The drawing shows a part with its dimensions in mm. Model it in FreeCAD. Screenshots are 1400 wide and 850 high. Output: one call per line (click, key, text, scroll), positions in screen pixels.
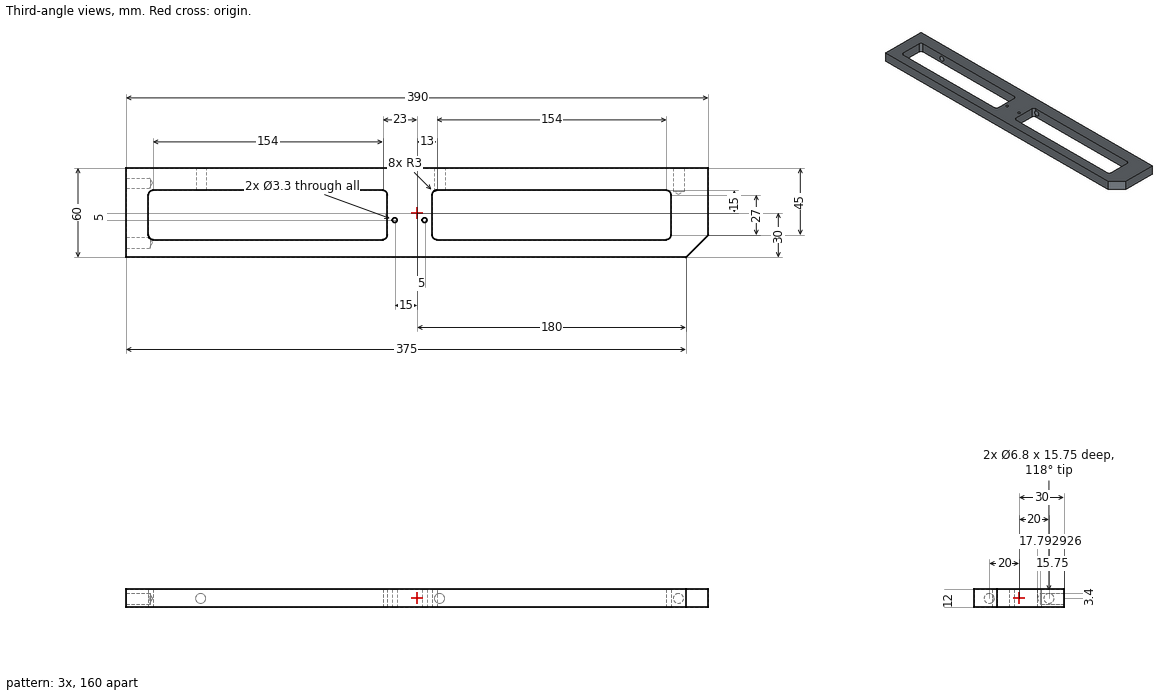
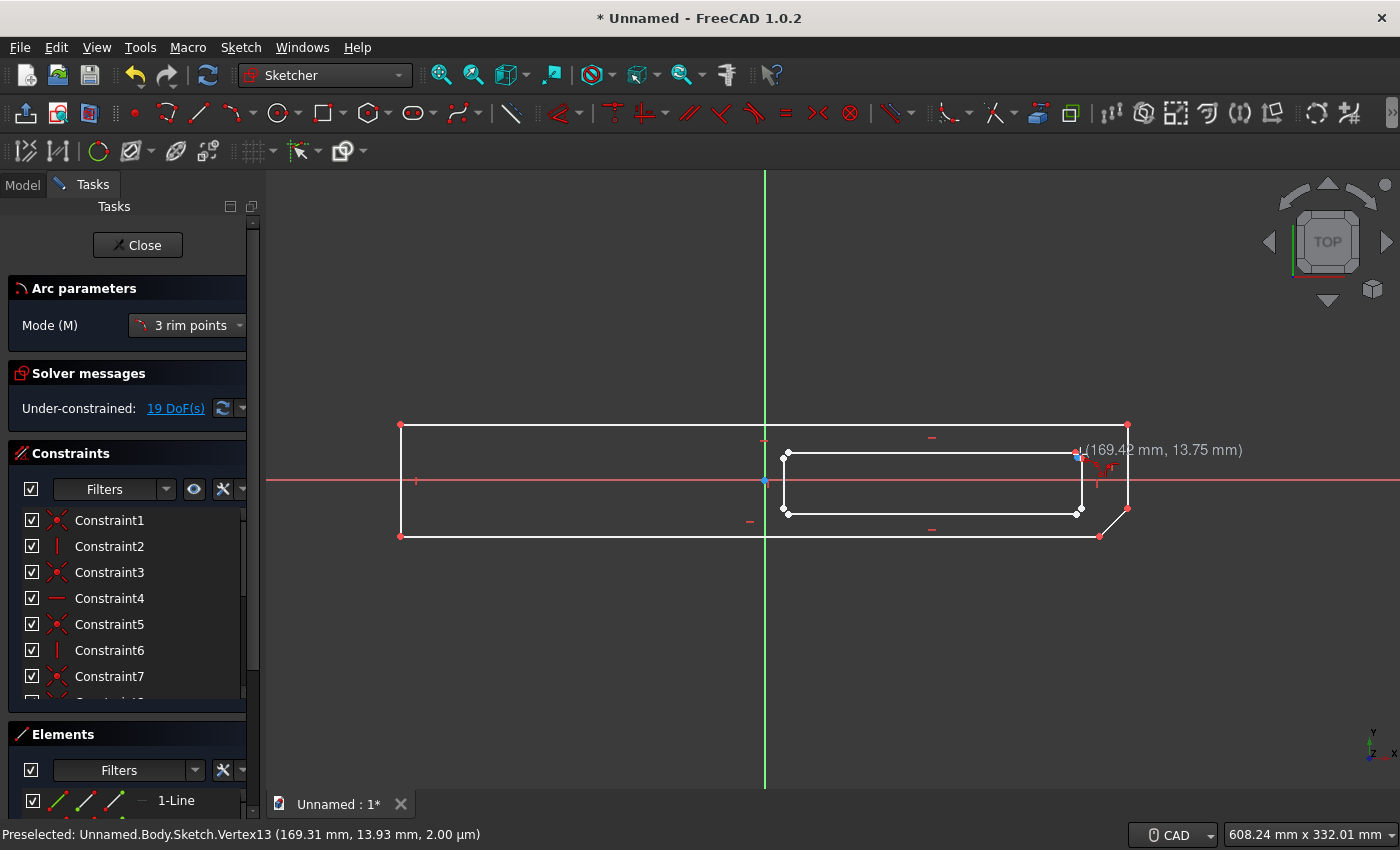
scroll(1082, 508, up, 4)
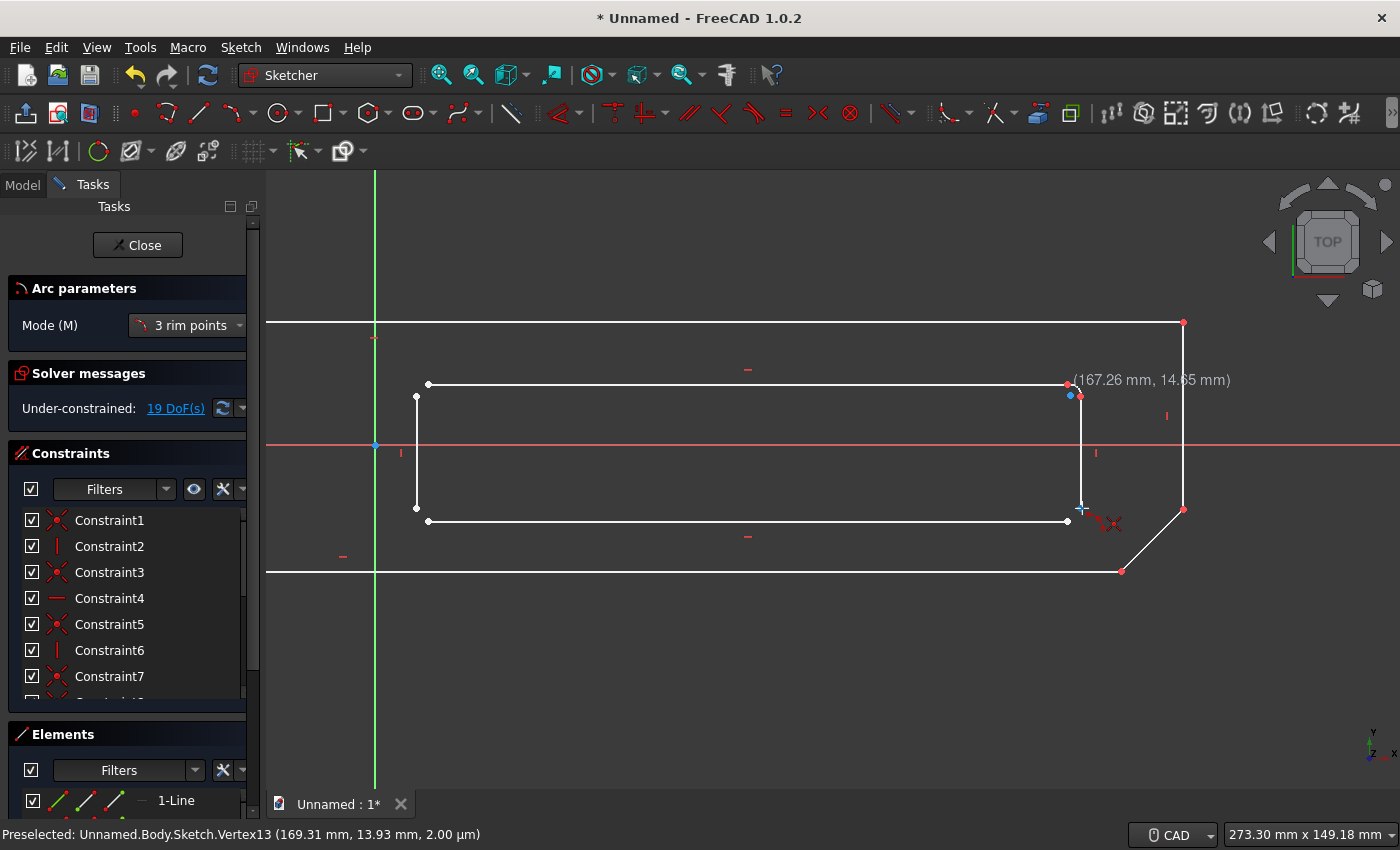
click(1081, 509)
click(1068, 522)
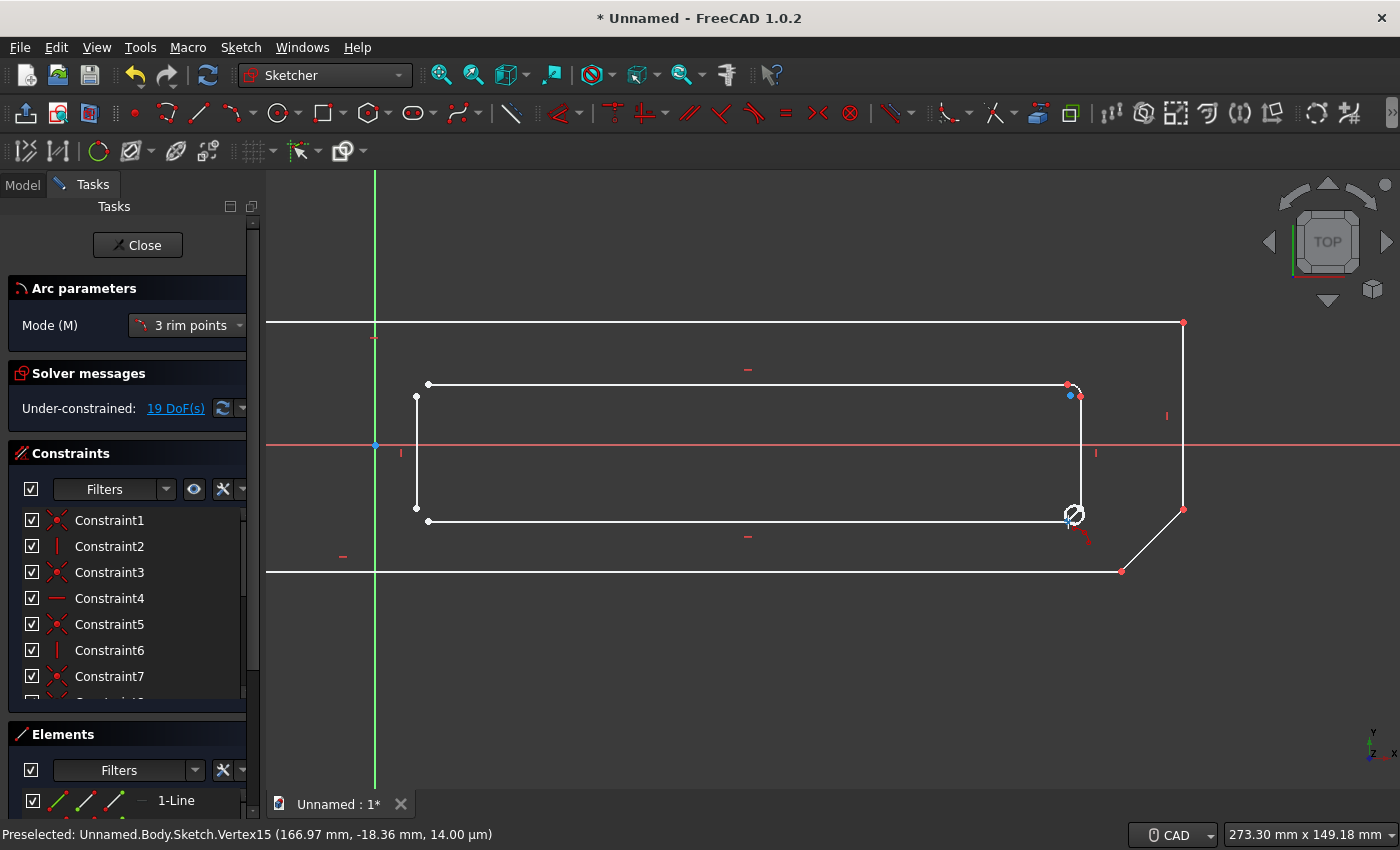
scroll(1077, 516, up, 8)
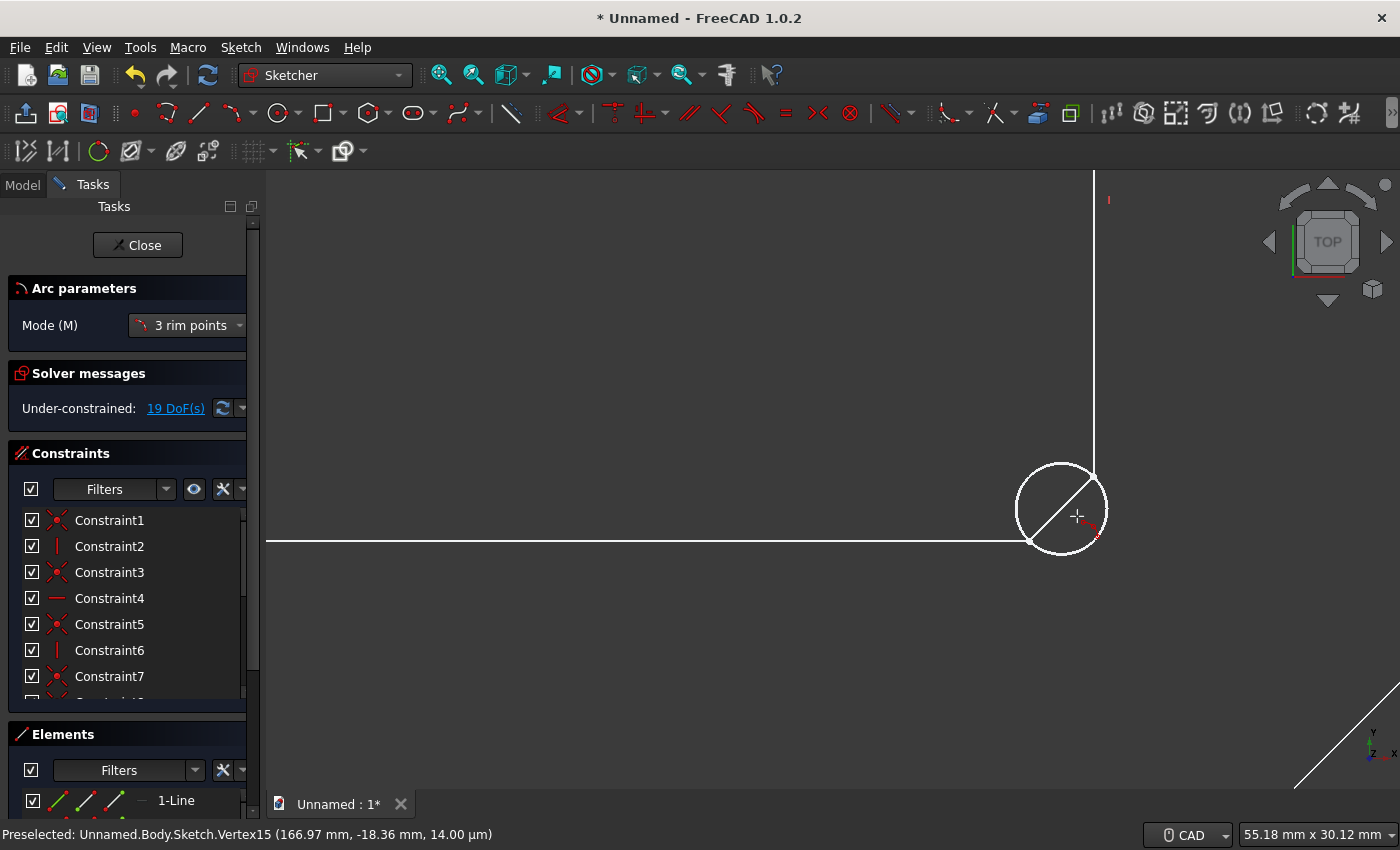
click(1074, 516)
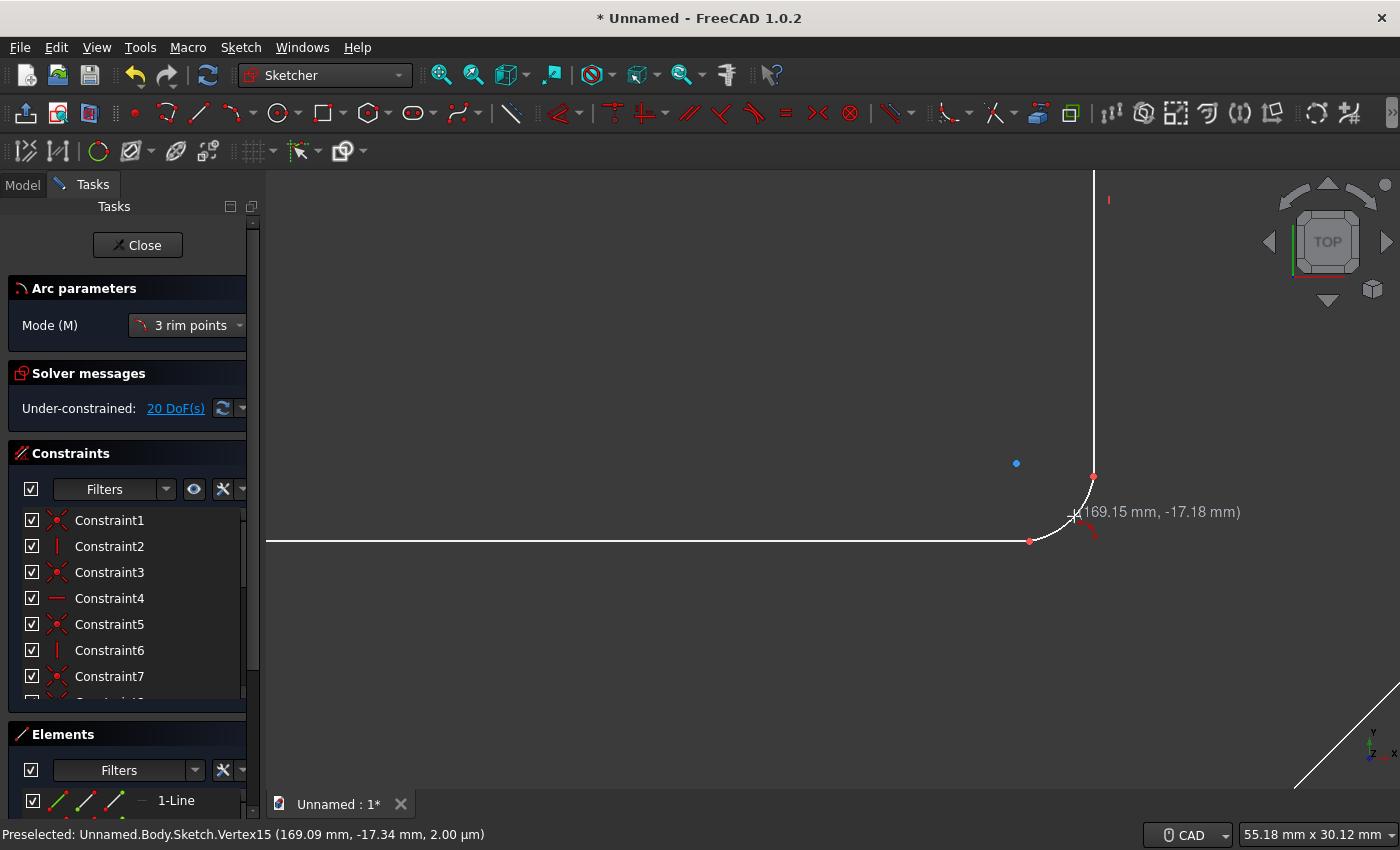
scroll(1080, 511, down, 12)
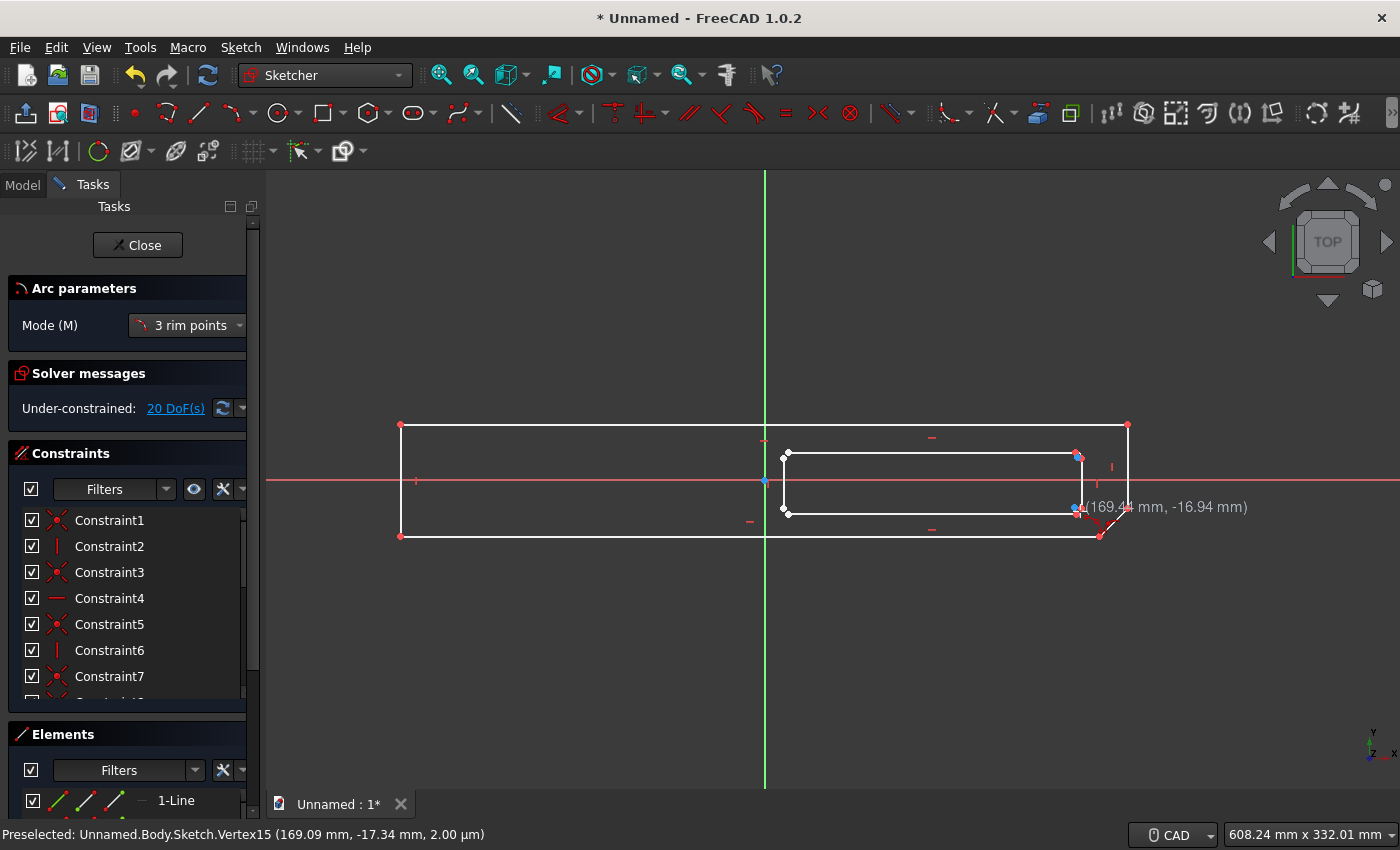
scroll(789, 514, up, 4)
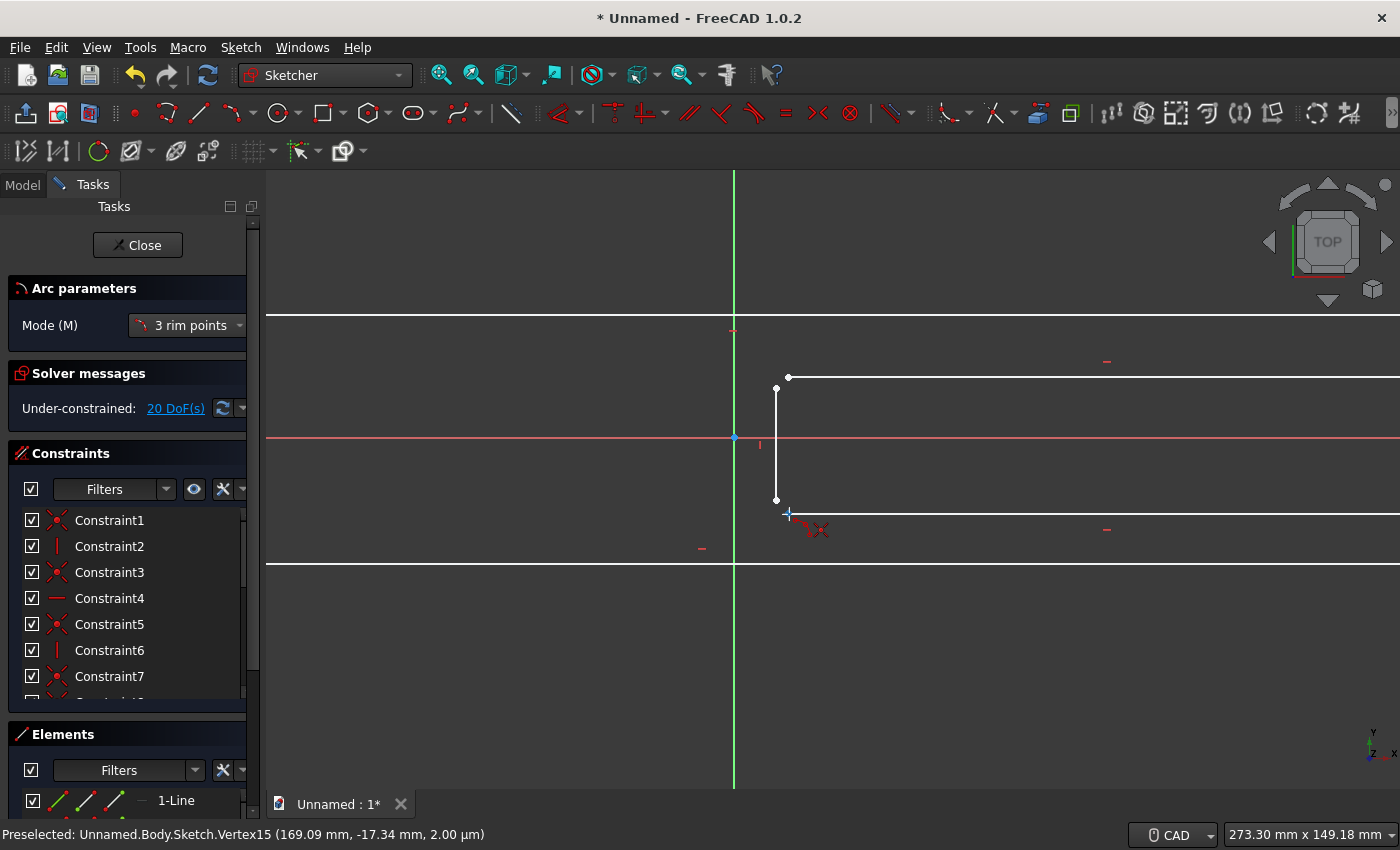
click(788, 514)
click(776, 501)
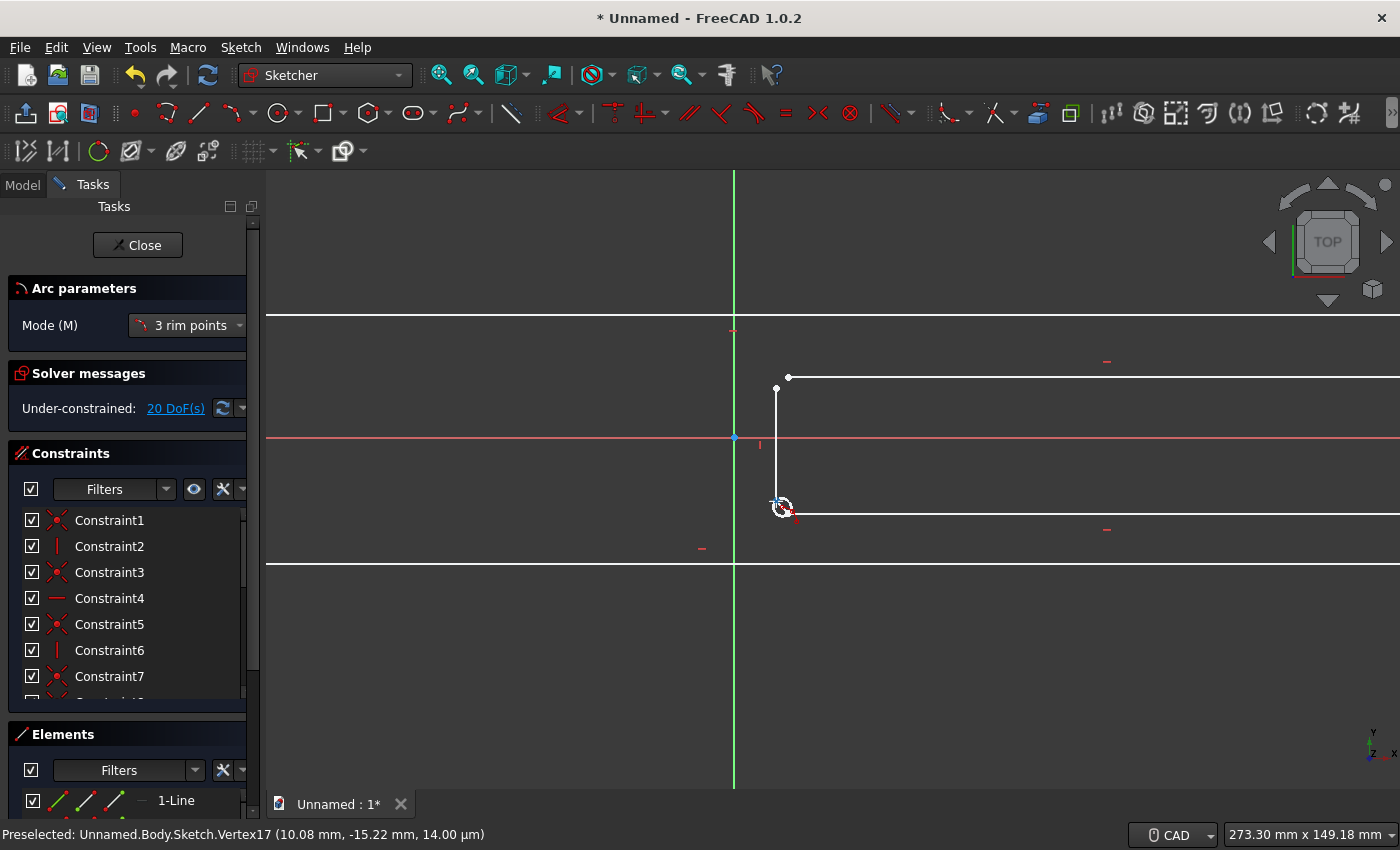
scroll(780, 509, up, 8)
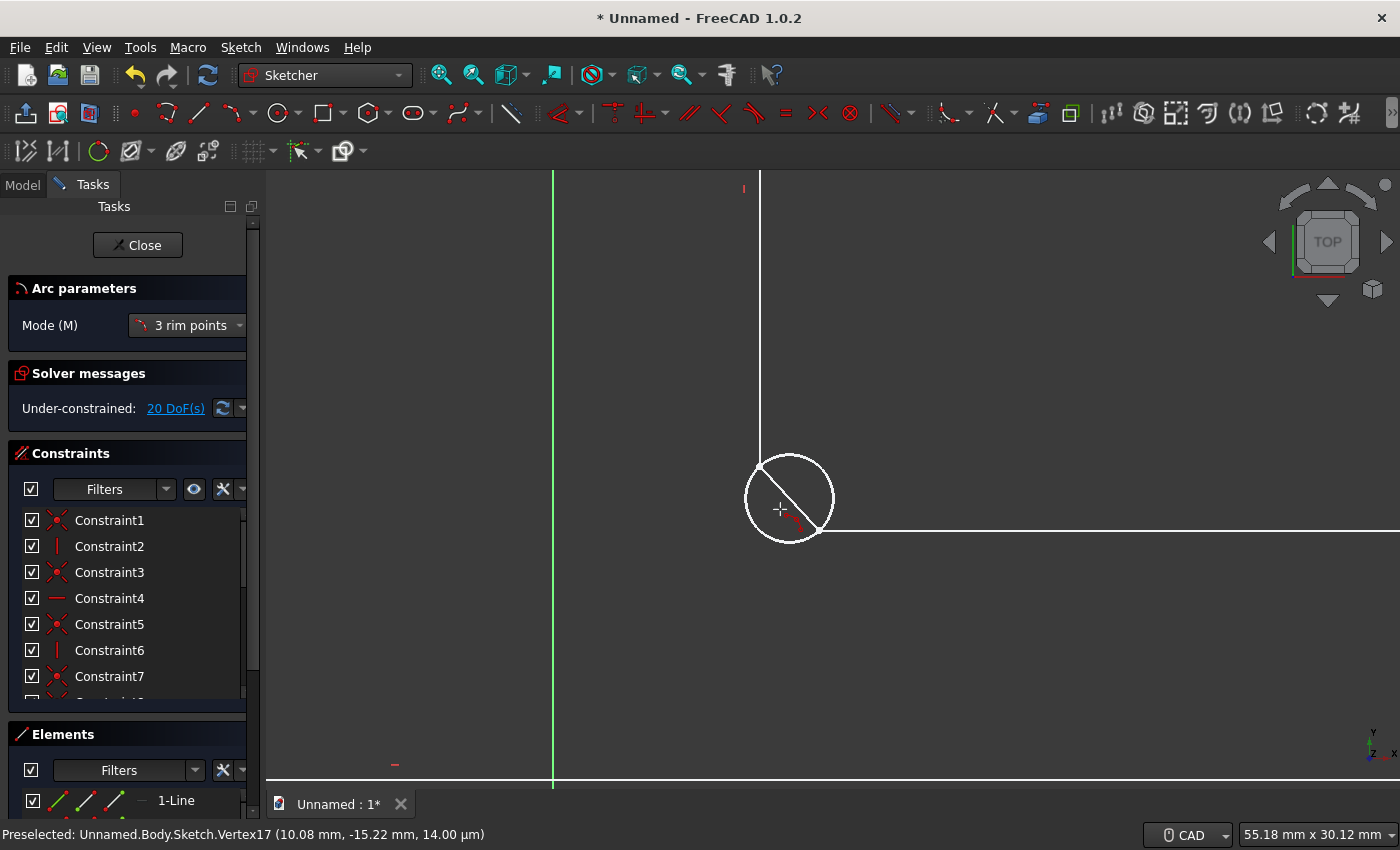
click(776, 505)